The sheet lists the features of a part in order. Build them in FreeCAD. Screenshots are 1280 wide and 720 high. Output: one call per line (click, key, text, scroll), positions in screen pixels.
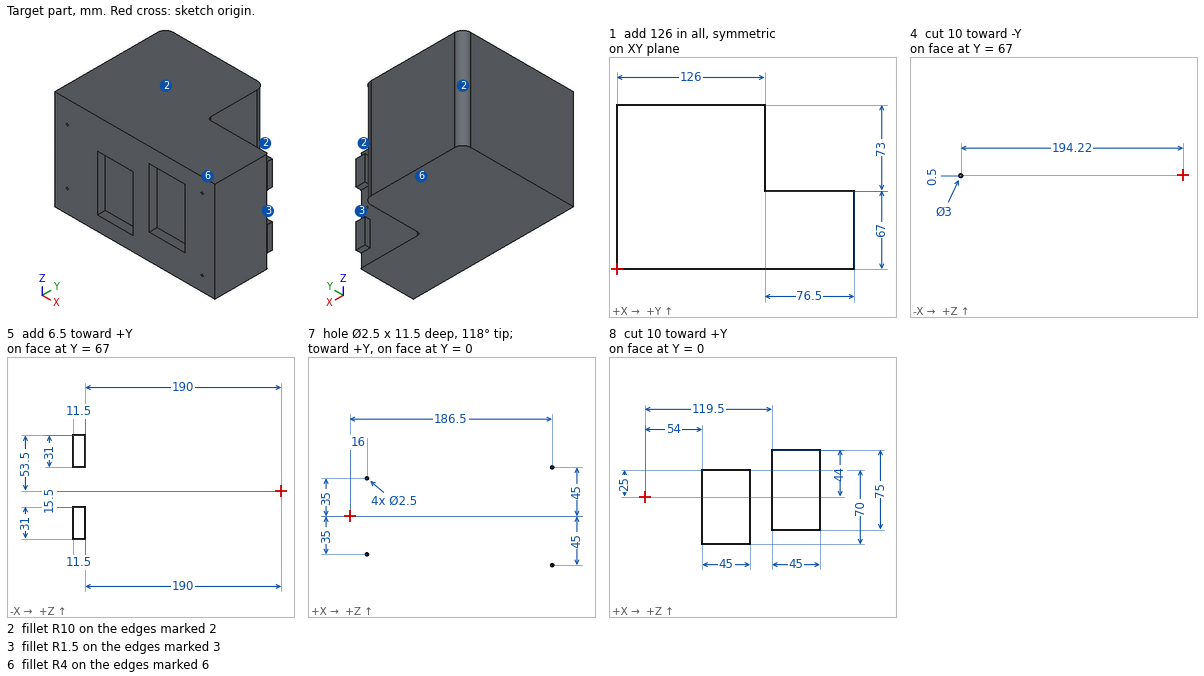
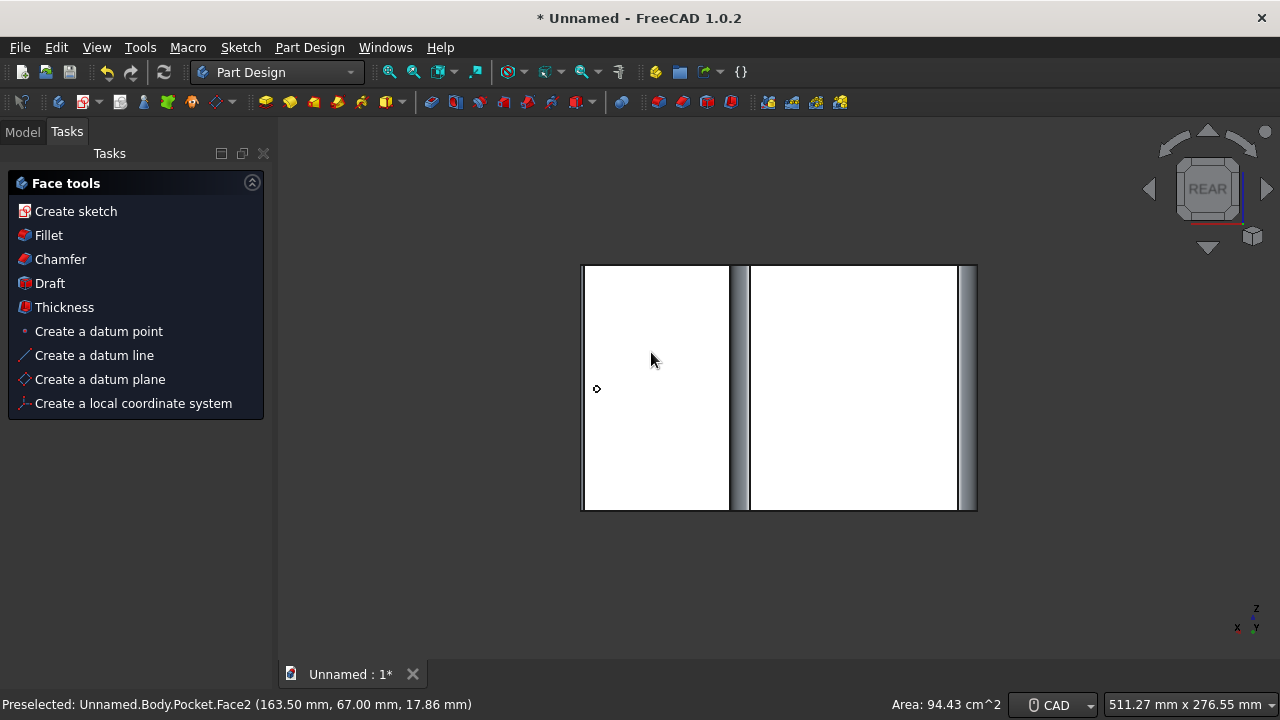
click(84, 102)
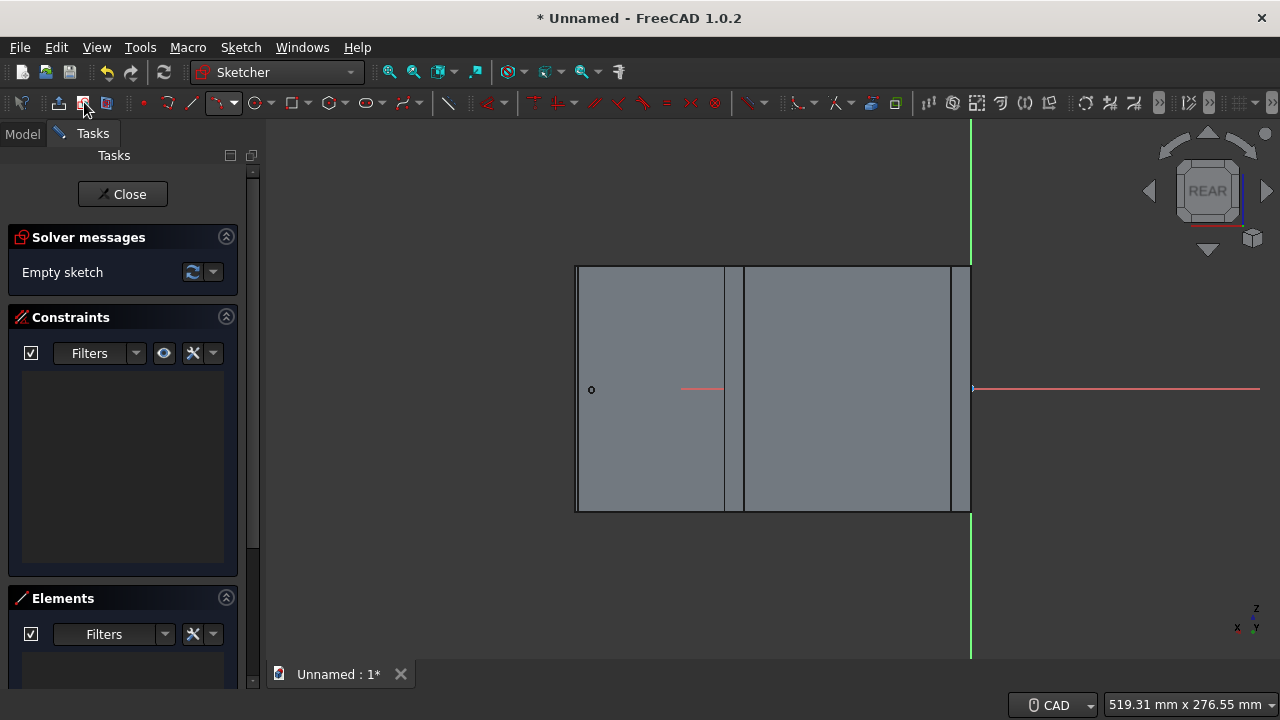
key(q)
key(s)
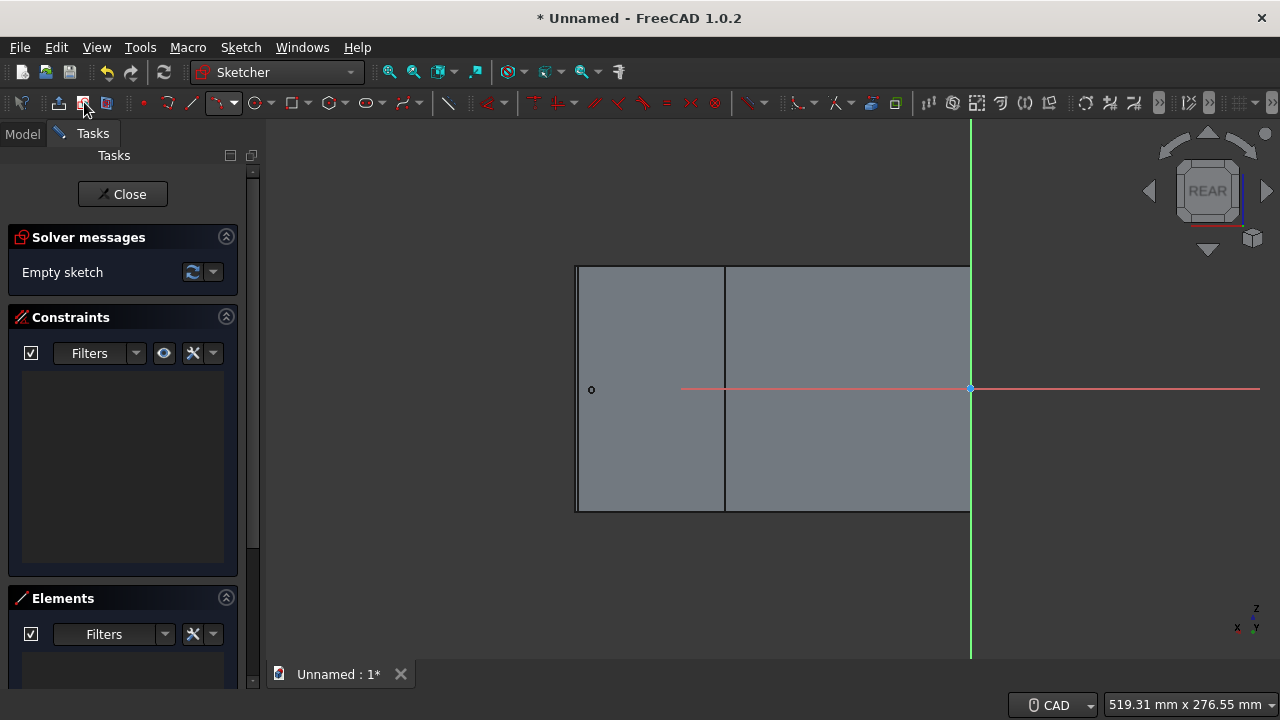
scroll(915, 368, up, 2)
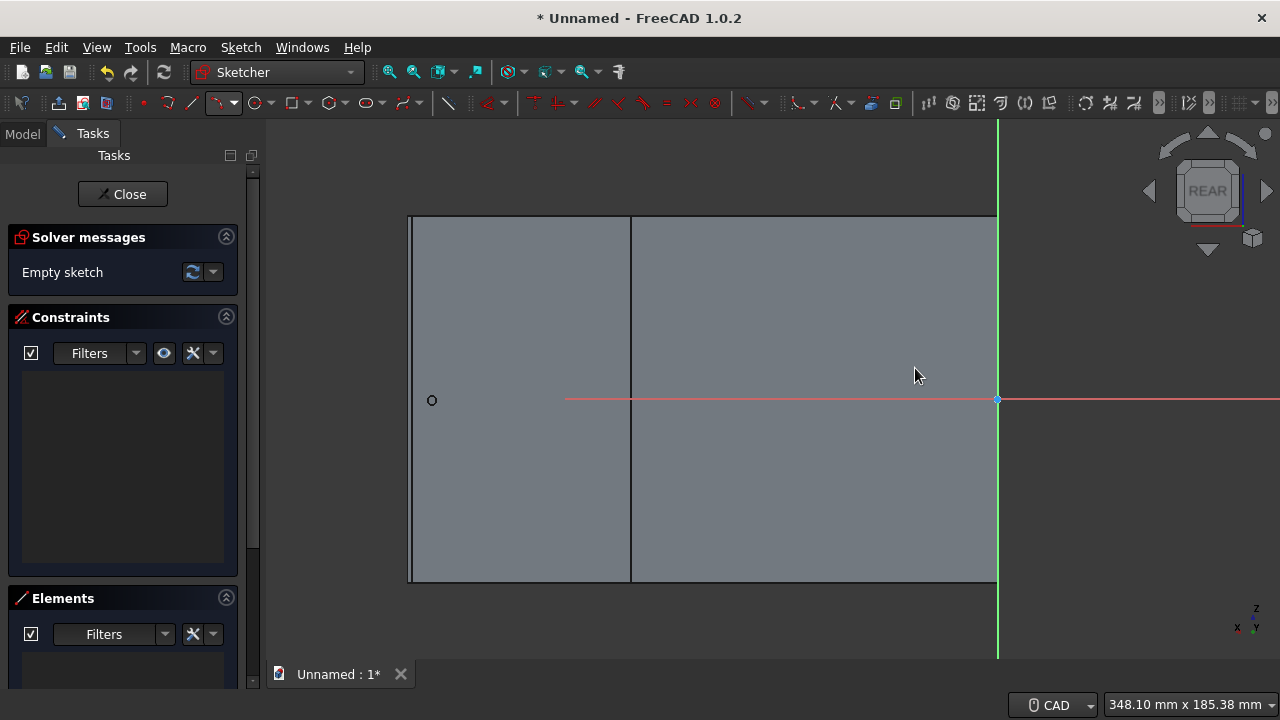
click(292, 104)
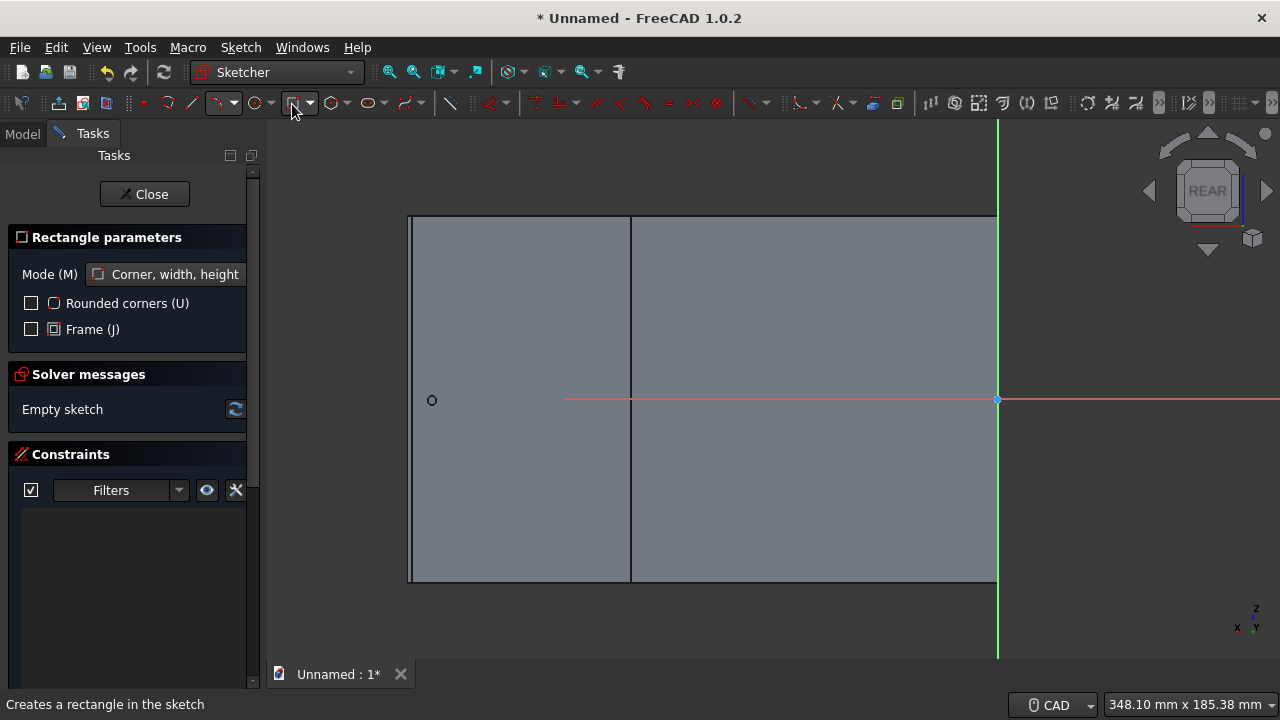
click(411, 243)
move(444, 334)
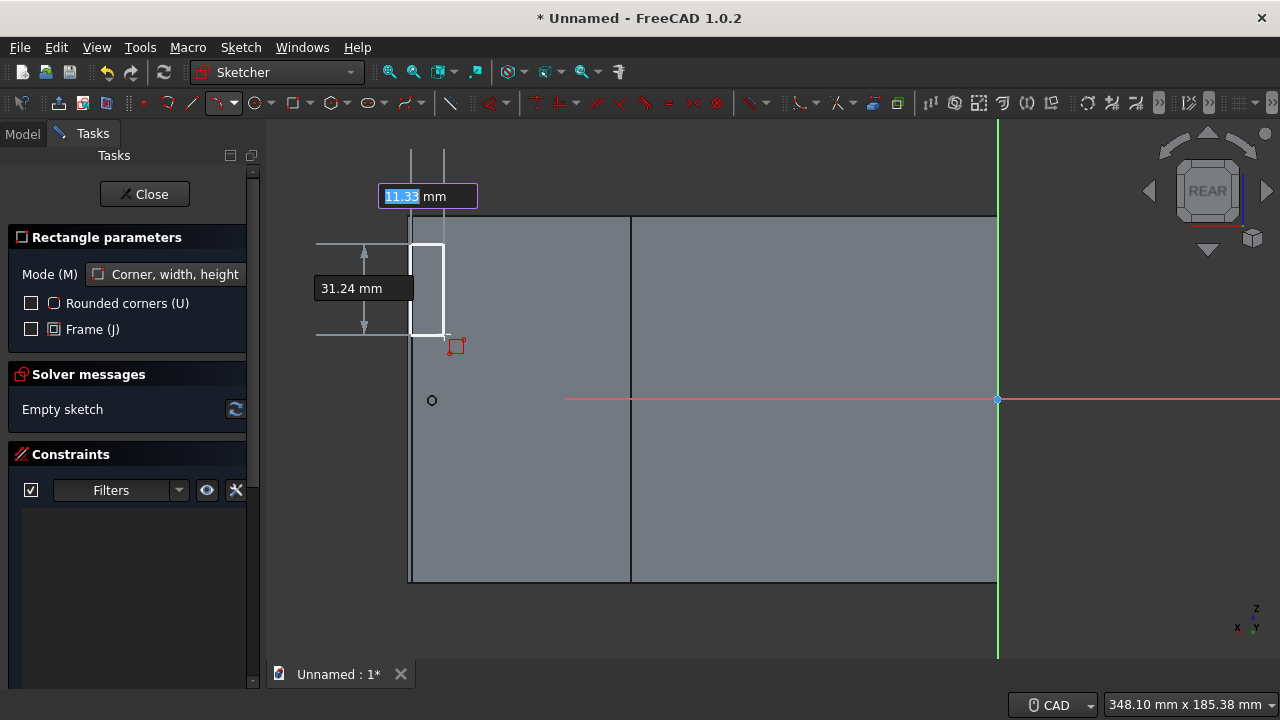
text(11.5)
key(Tab)
text(31)
key(Return)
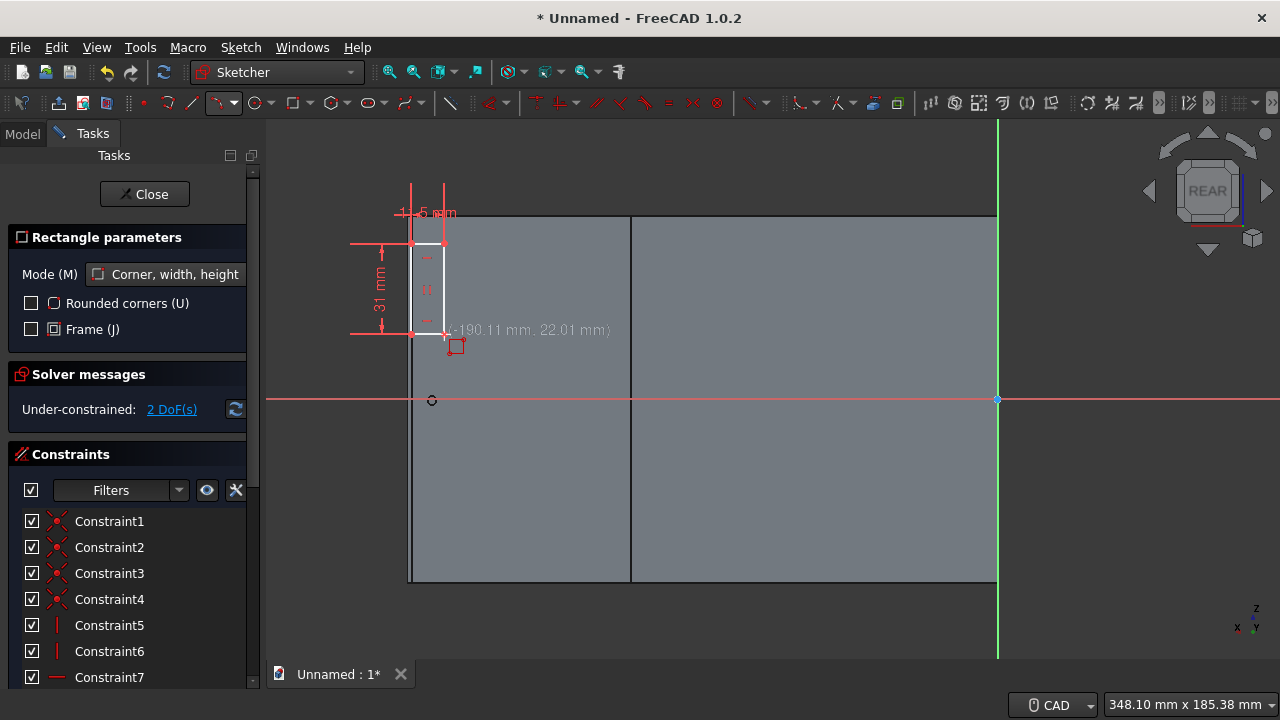
click(411, 444)
move(444, 535)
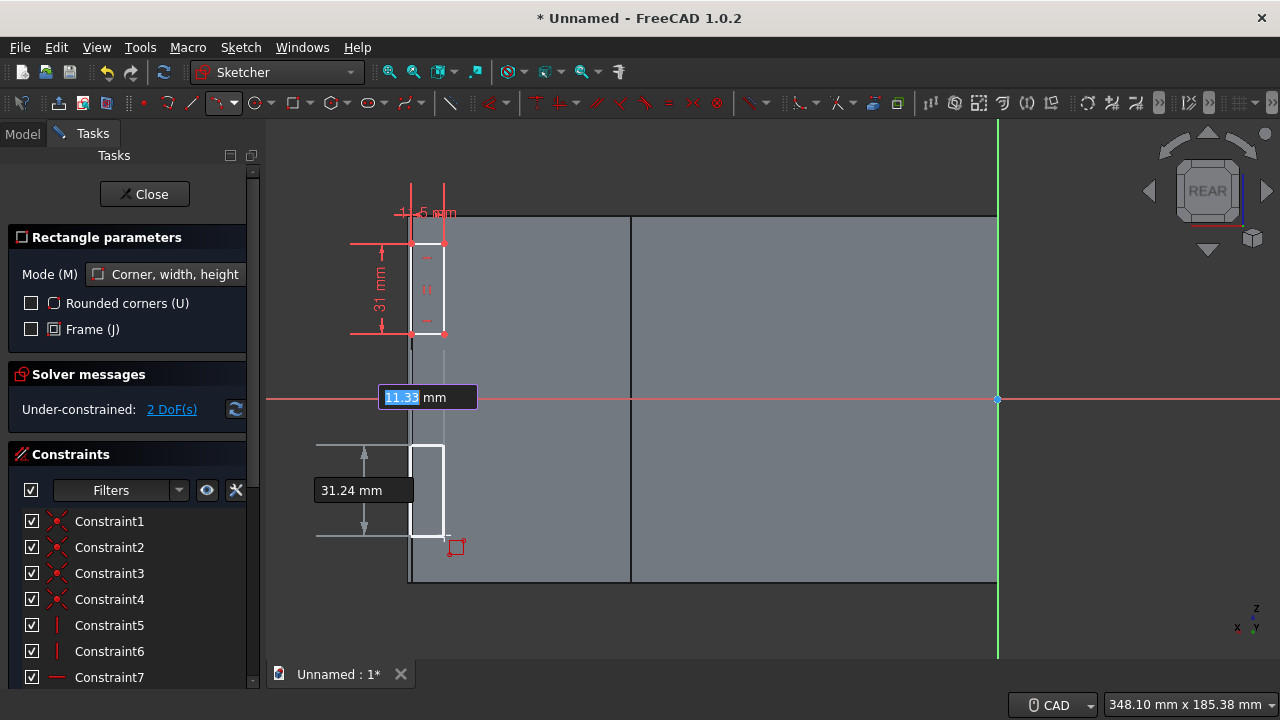
text(11.5)
key(Tab)
text(31)
key(Return)
key(Escape)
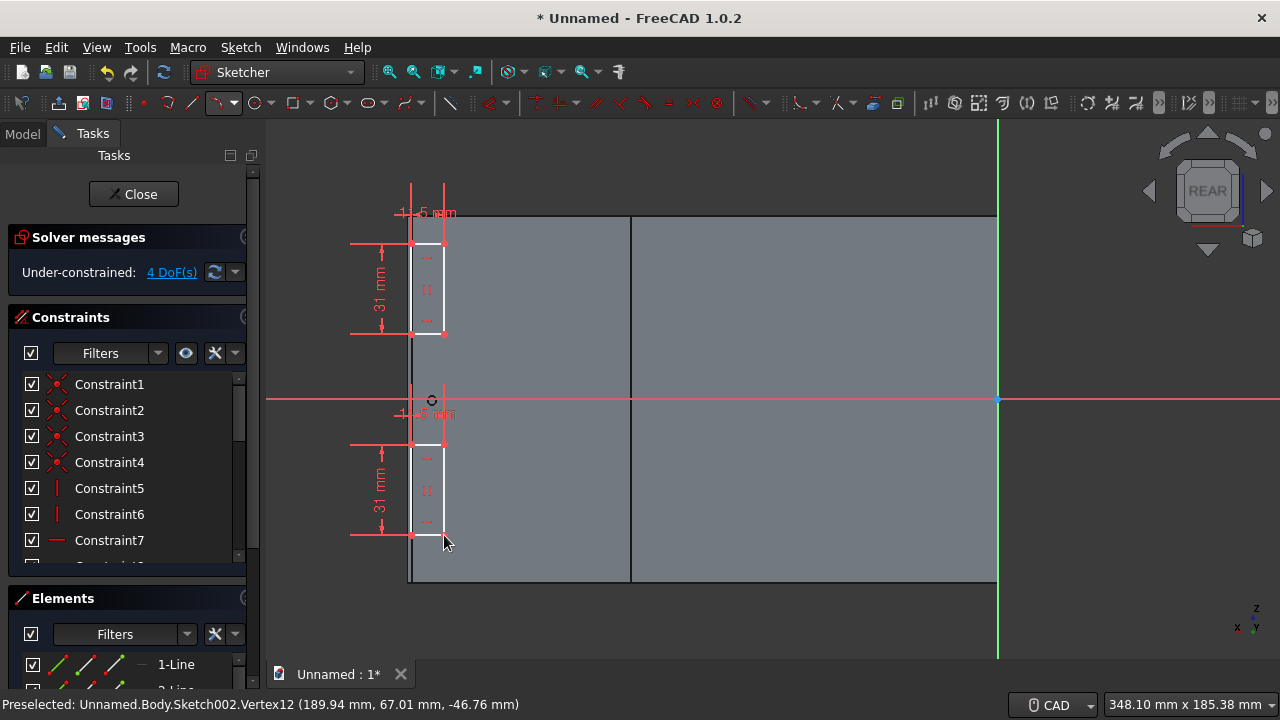
click(490, 104)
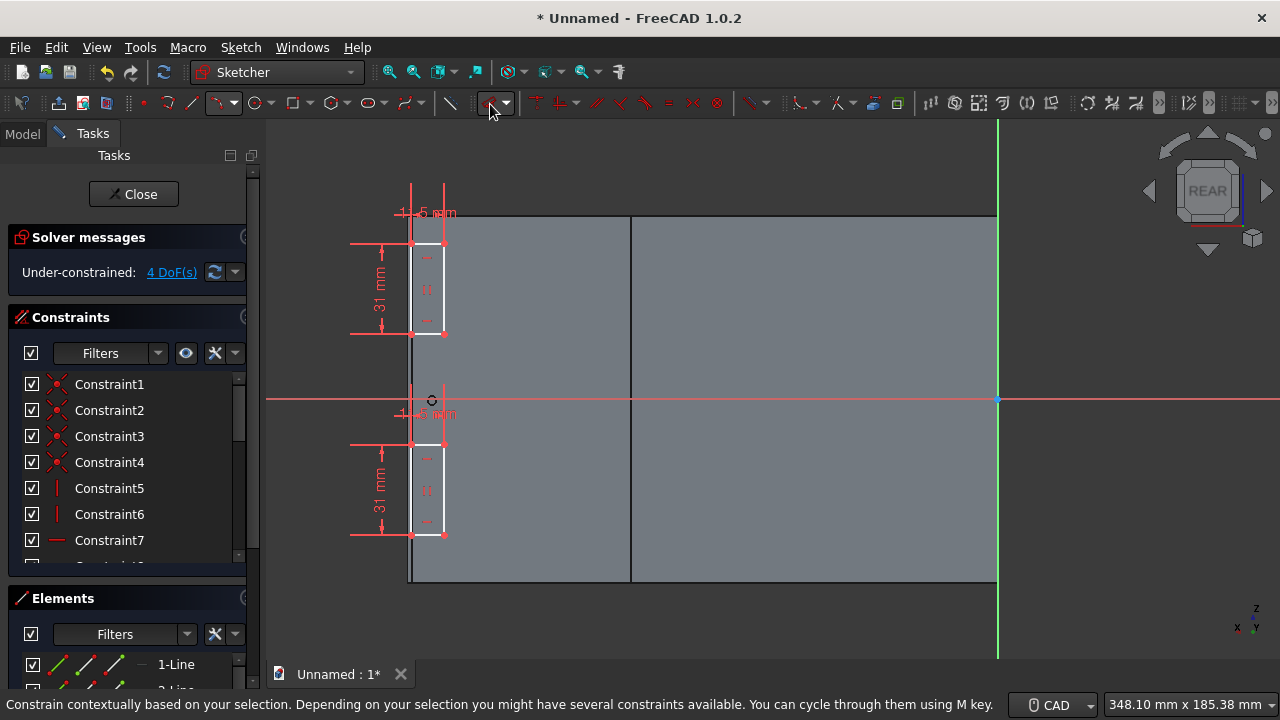
click(444, 334)
click(721, 300)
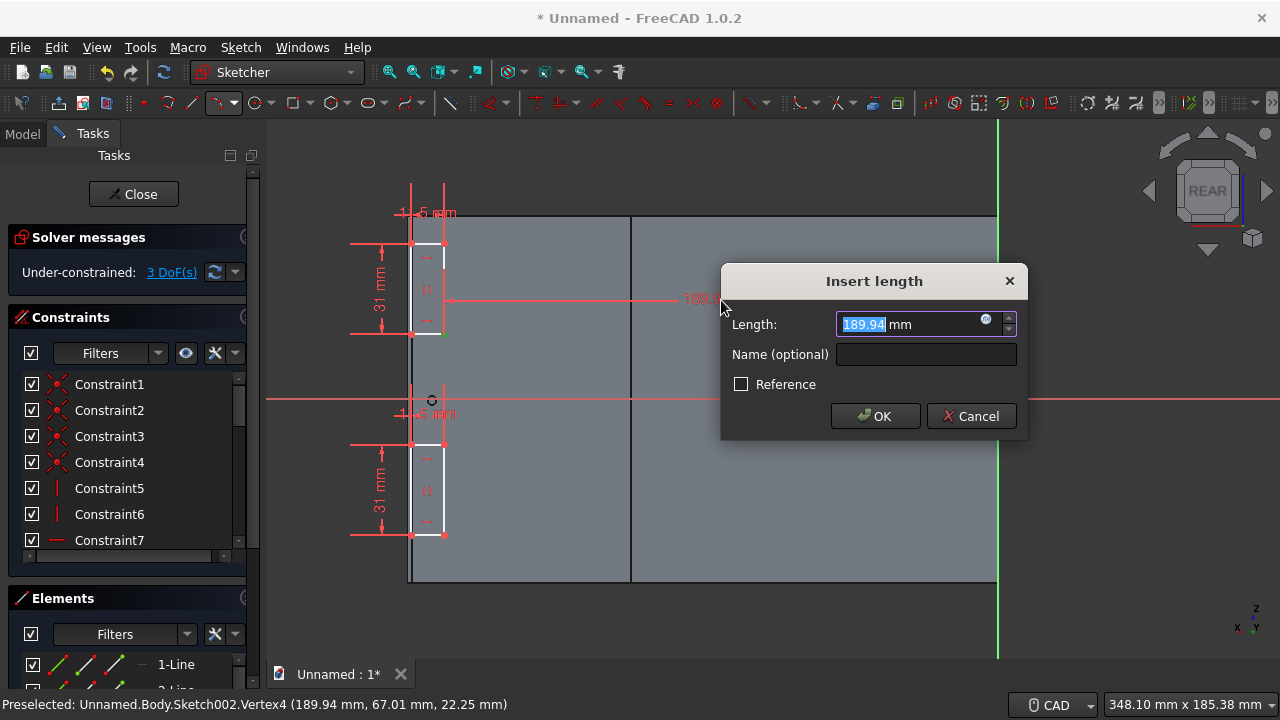
text(190)
key(Return)